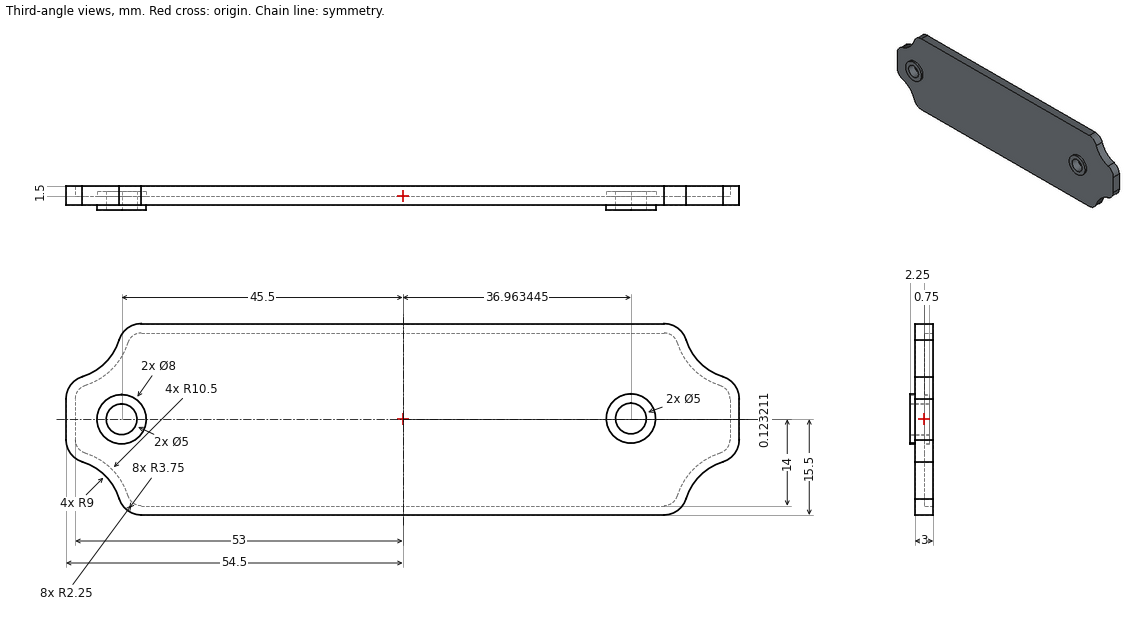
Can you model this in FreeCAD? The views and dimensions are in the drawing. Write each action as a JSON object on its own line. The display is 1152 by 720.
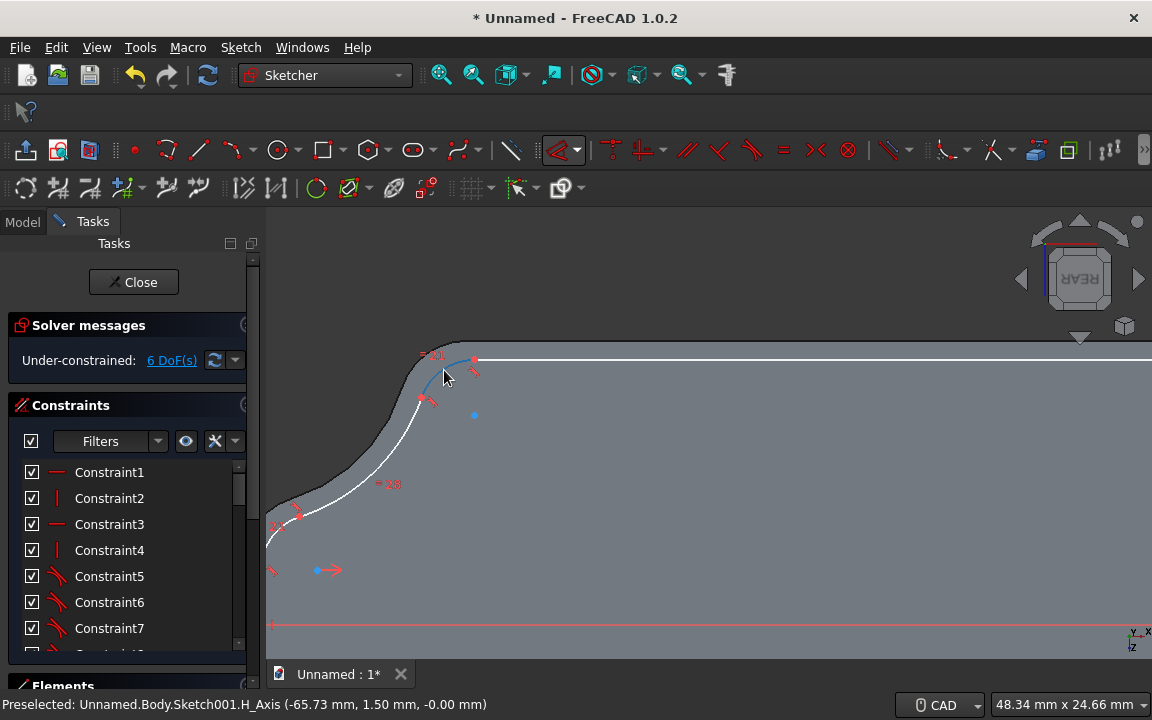
{"action": "left_click", "coordinate": [442, 370]}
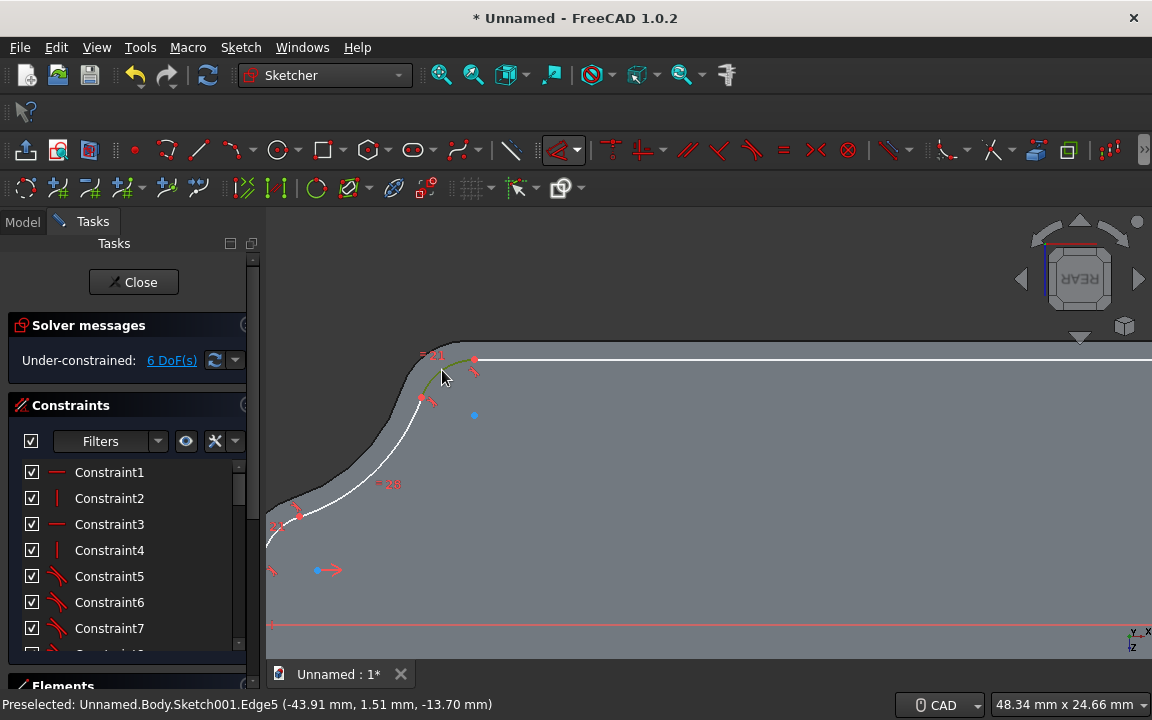
{"action": "left_click", "coordinate": [580, 150]}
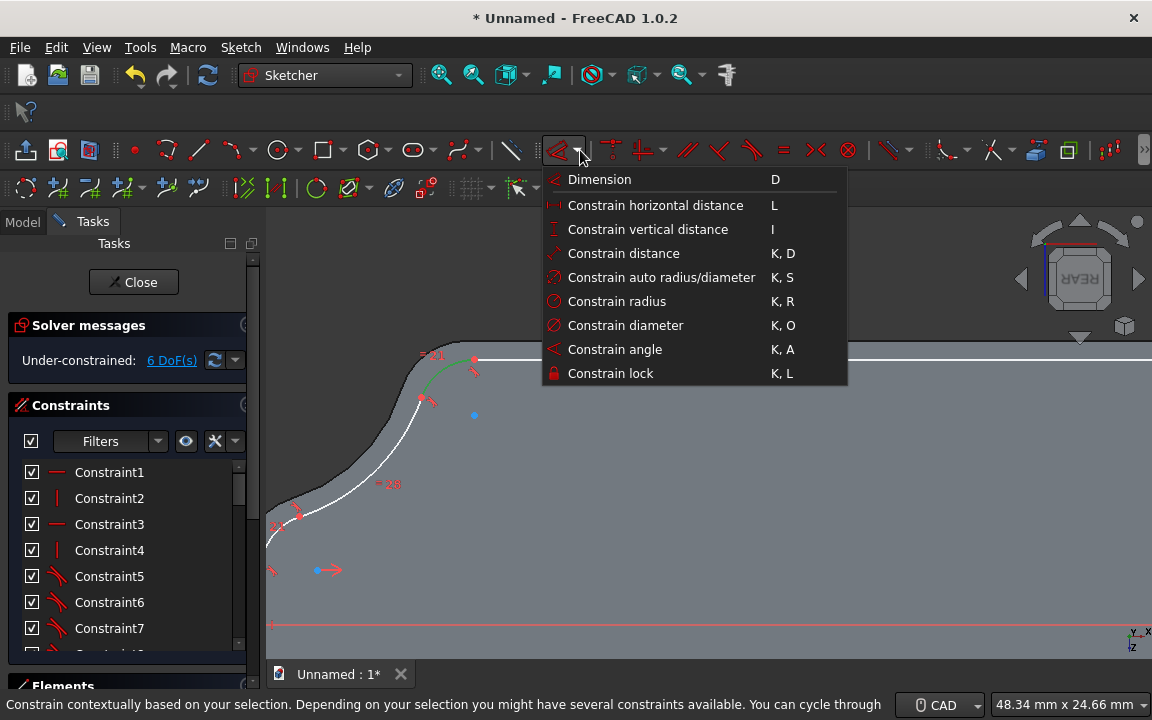
{"action": "left_click", "coordinate": [695, 301]}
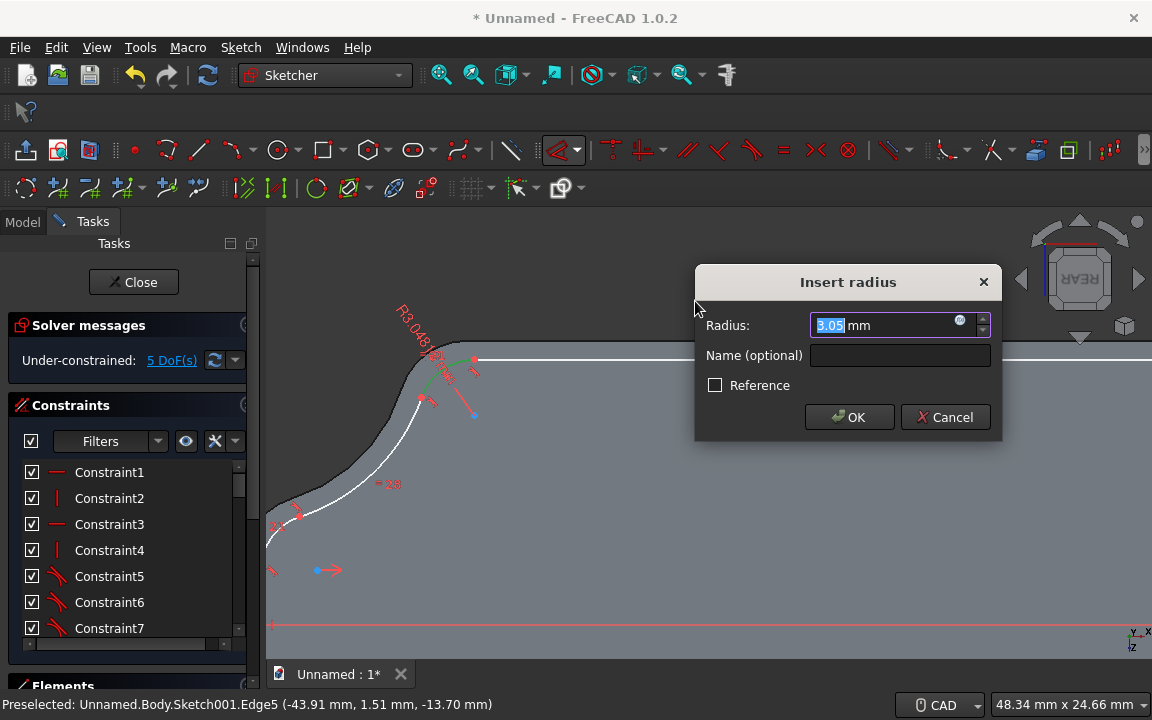
{"action": "type", "text": "2.25"}
{"action": "key", "text": "Return"}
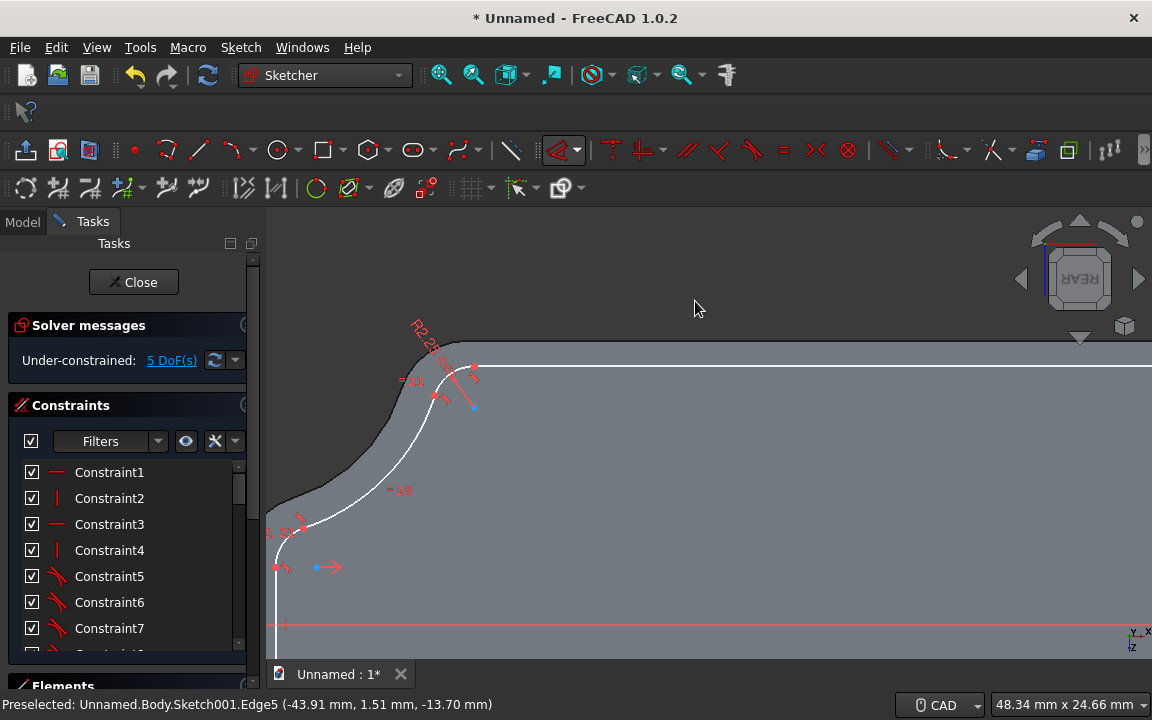
{"action": "scroll", "coordinate": [443, 370], "scroll_direction": "down", "scroll_amount": 7}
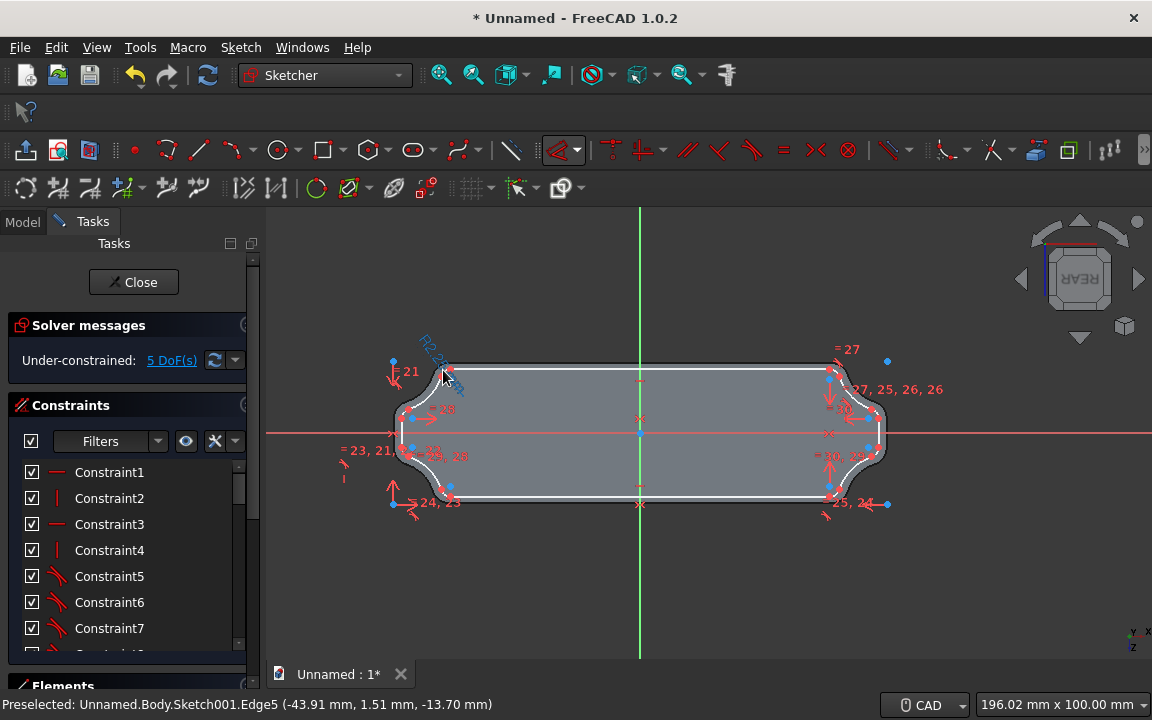
{"action": "left_click", "coordinate": [422, 403]}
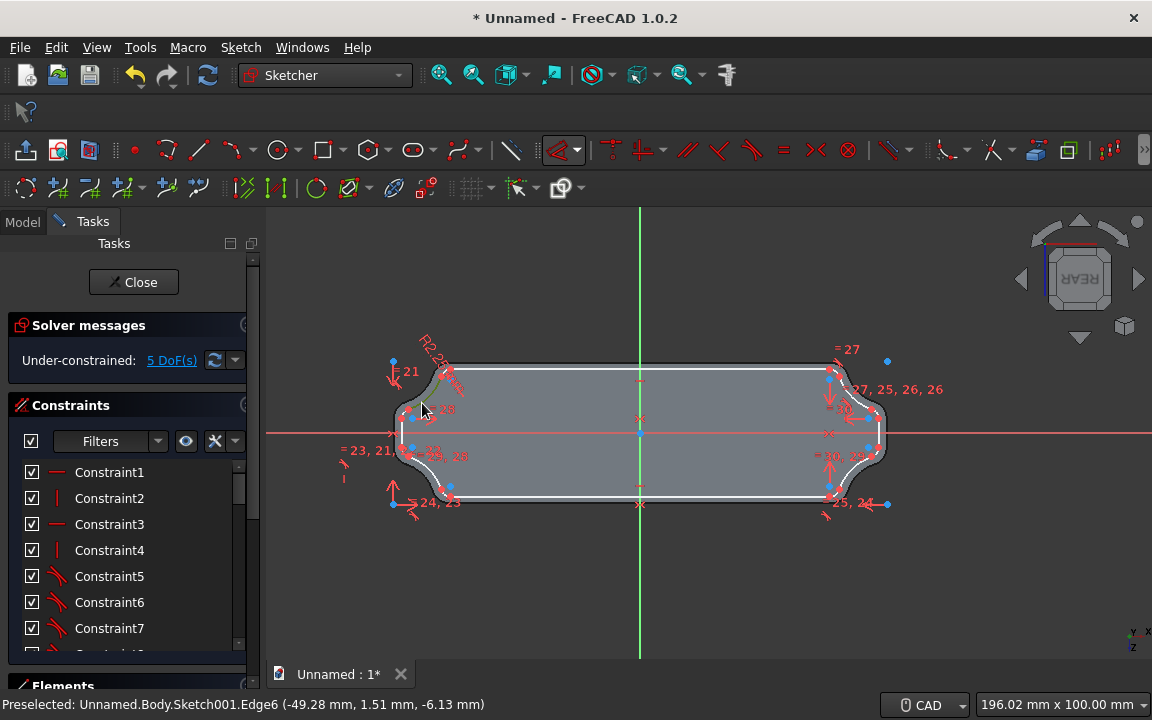
{"action": "key", "text": "k r"}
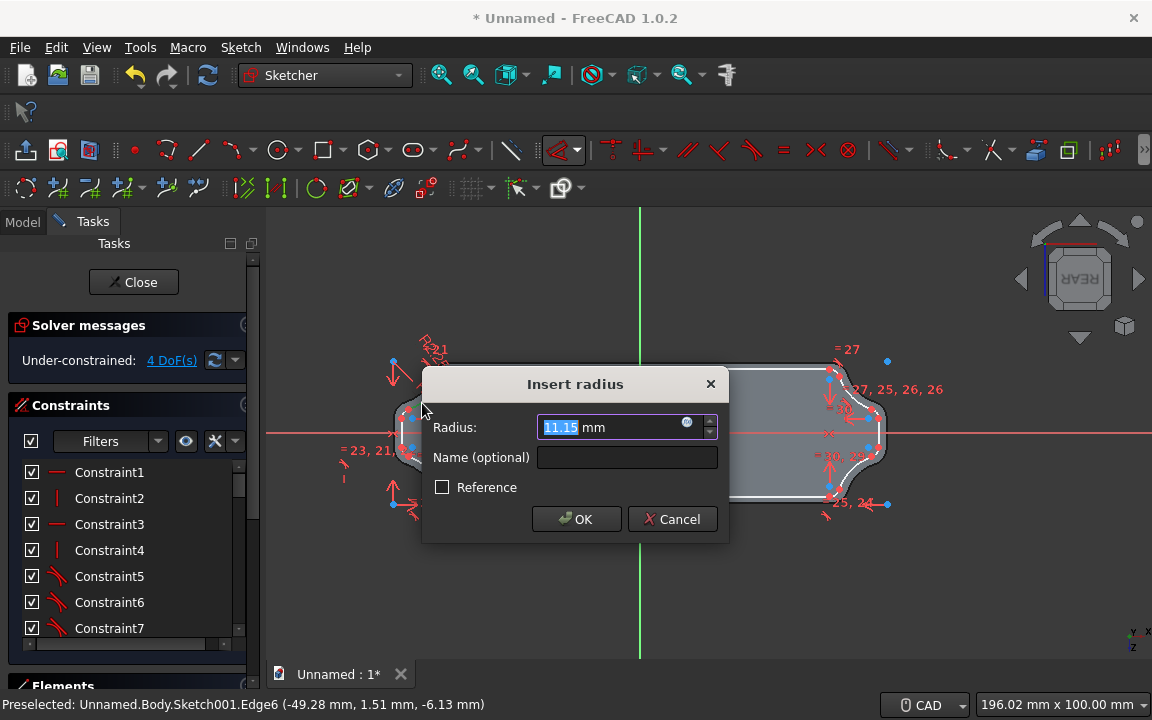
{"action": "type", "text": "10.5"}
{"action": "key", "text": "Return"}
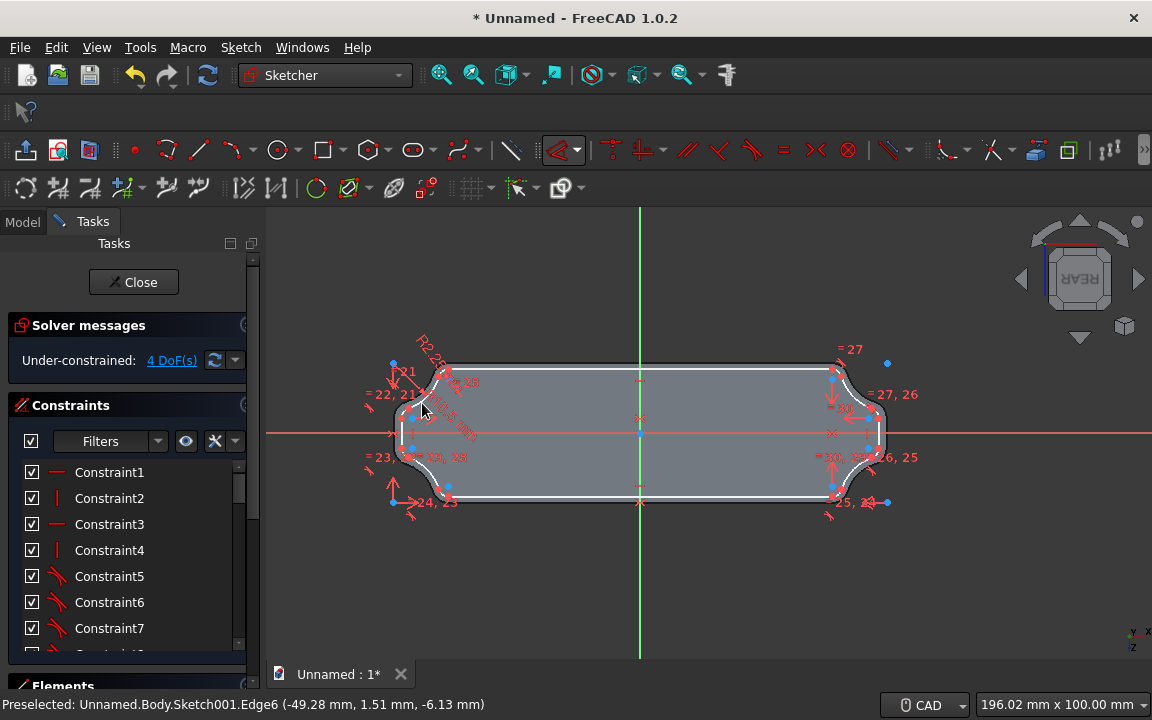
{"action": "left_click", "coordinate": [832, 369]}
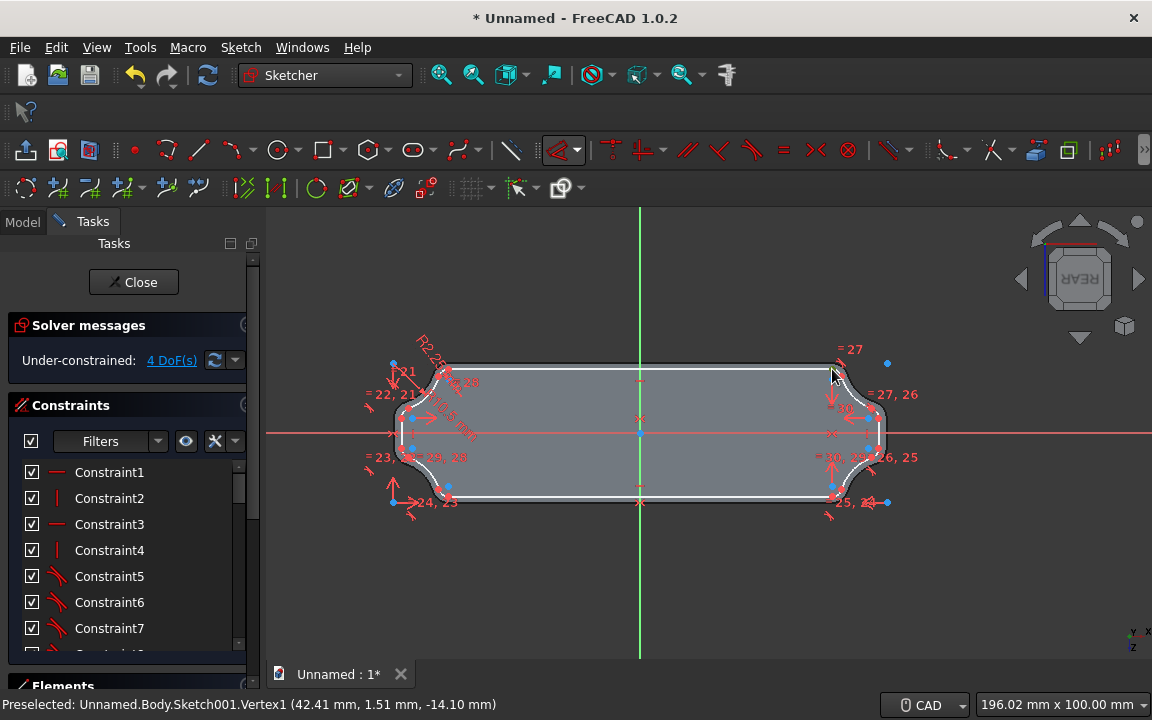
{"action": "left_click", "coordinate": [580, 150]}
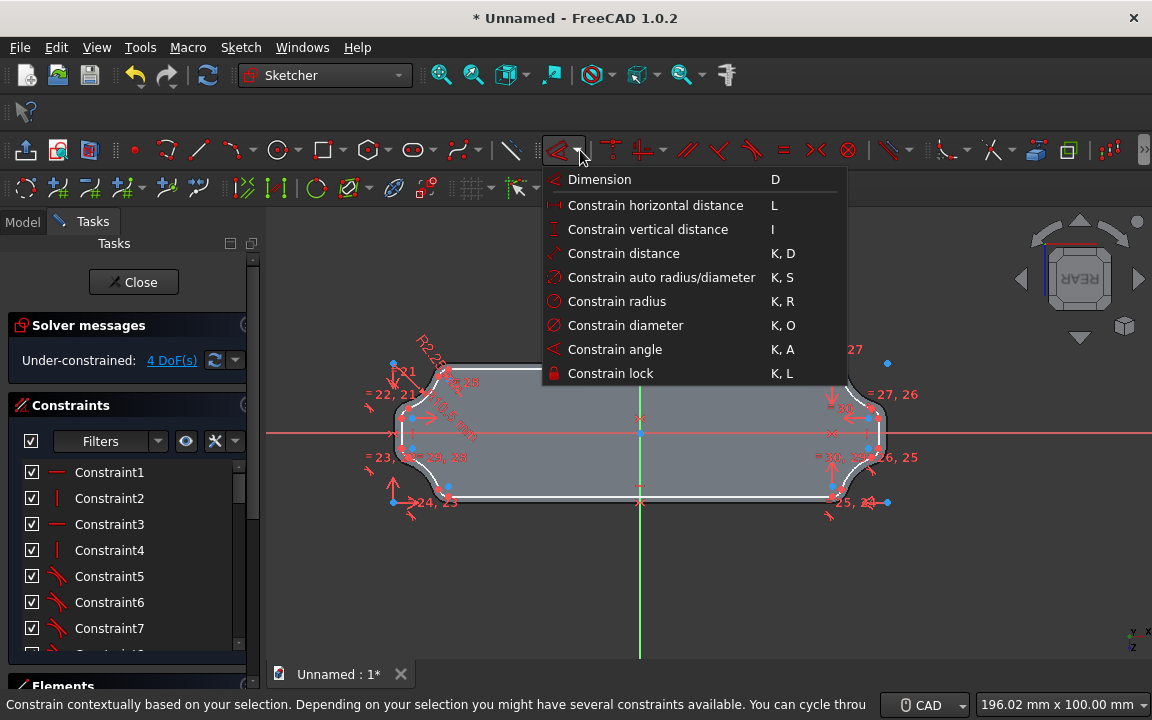
{"action": "left_click", "coordinate": [695, 229]}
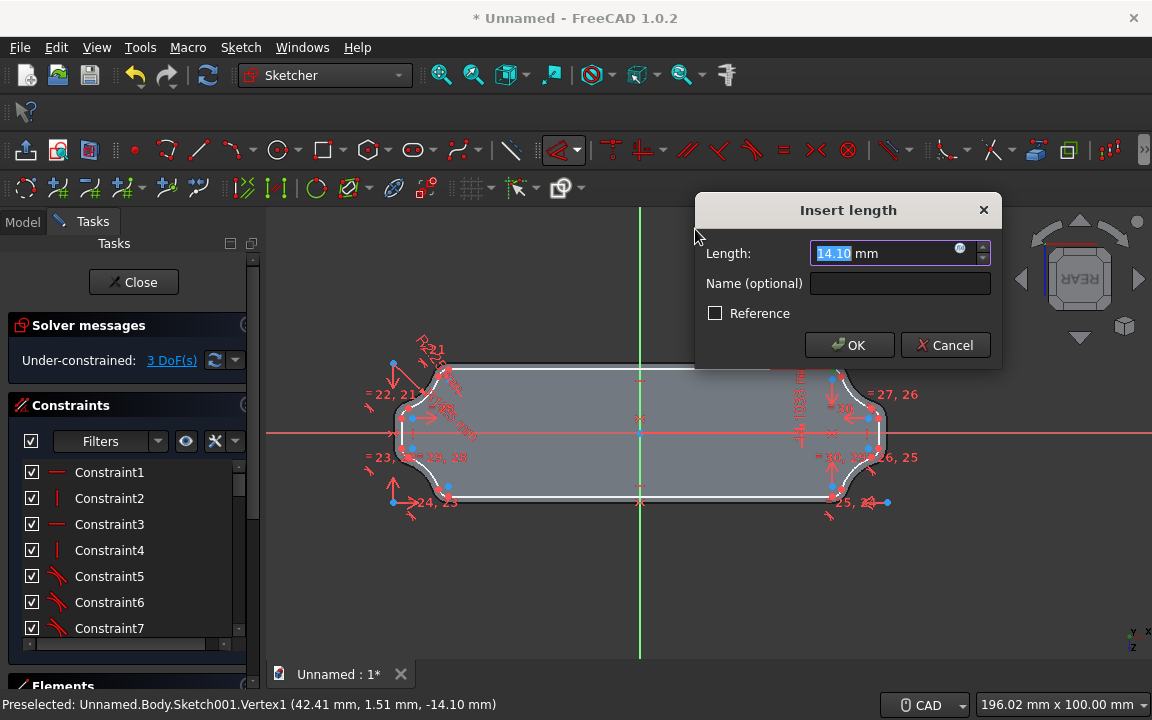
{"action": "type", "text": "14"}
{"action": "key", "text": "Return"}